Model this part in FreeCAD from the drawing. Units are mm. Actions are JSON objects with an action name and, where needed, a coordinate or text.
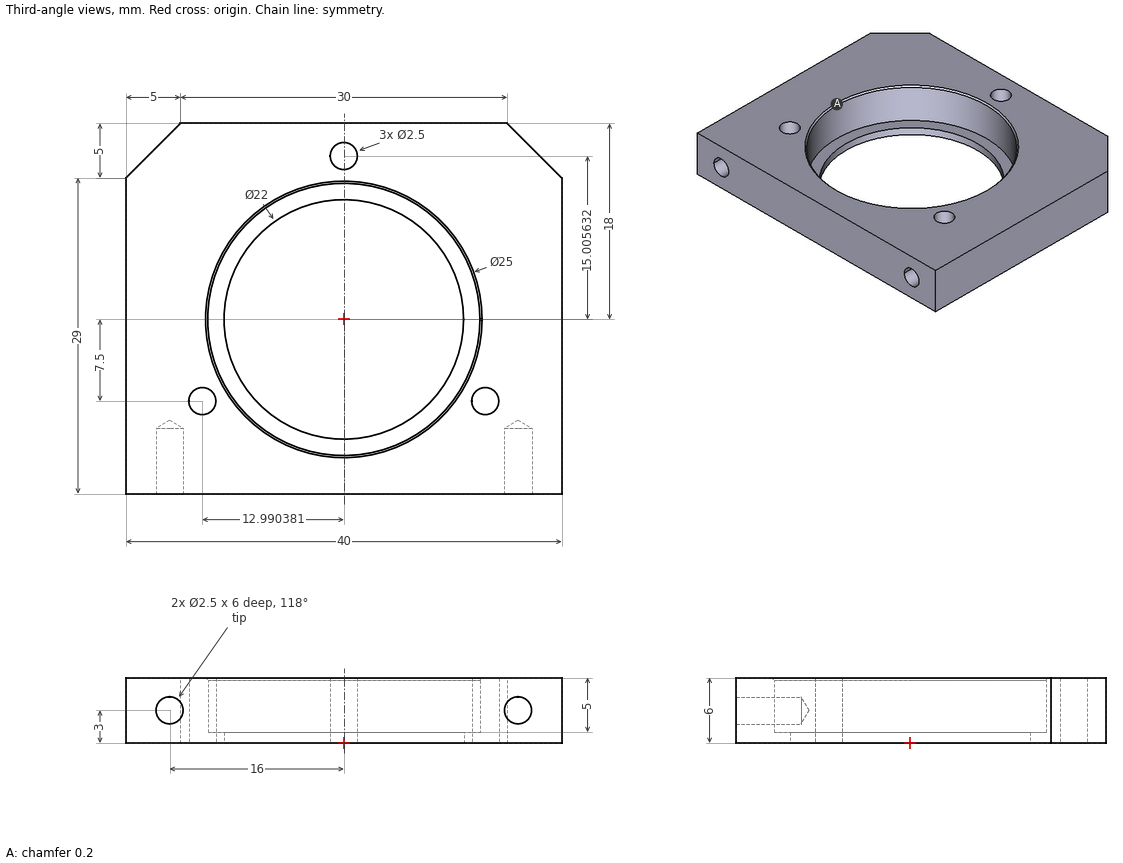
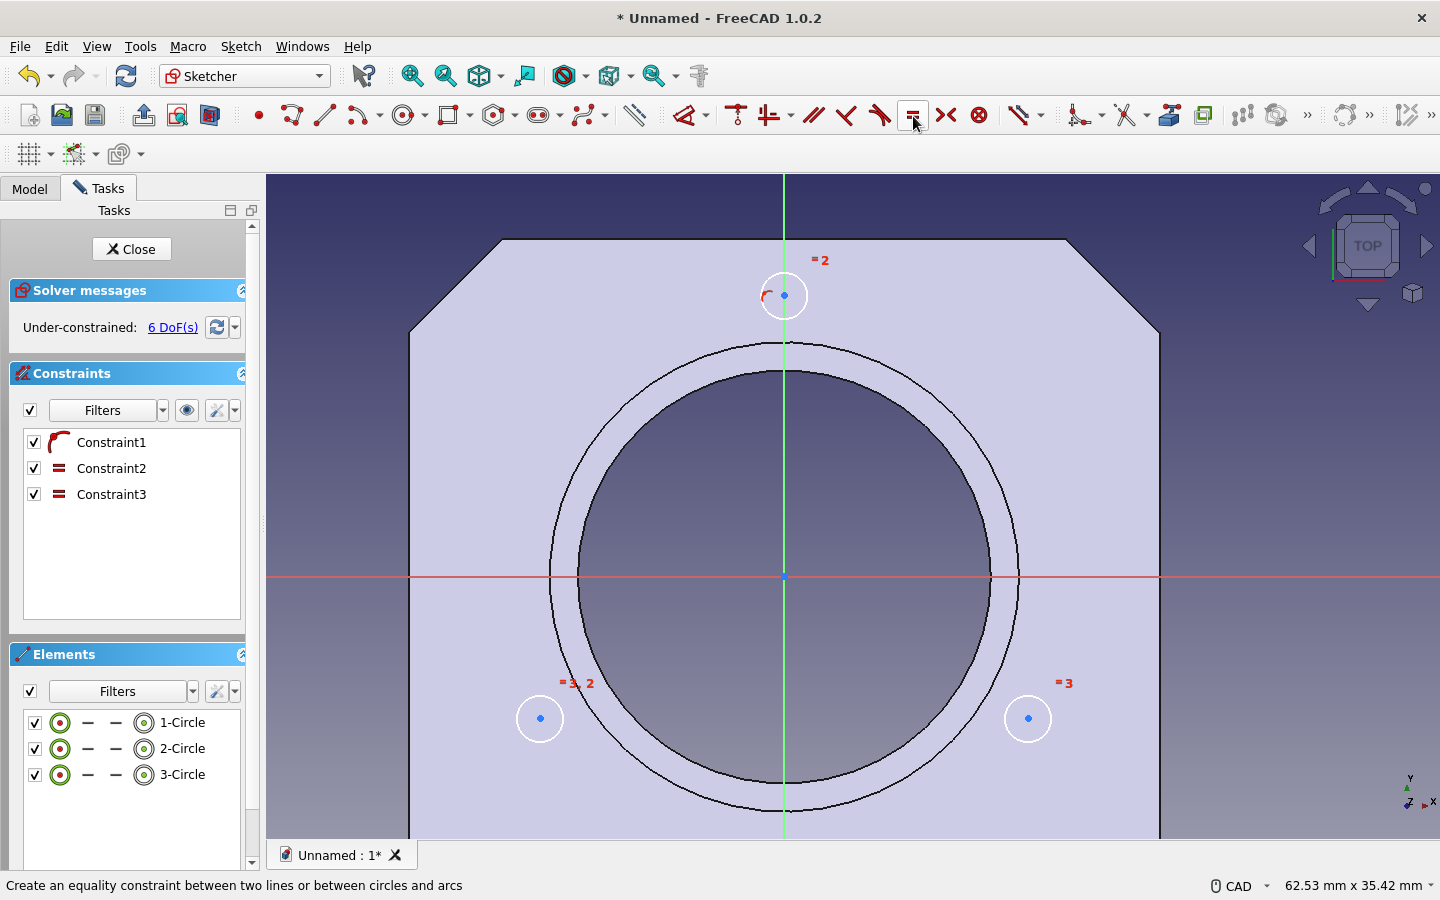
{"action": "left_click", "coordinate": [540, 719]}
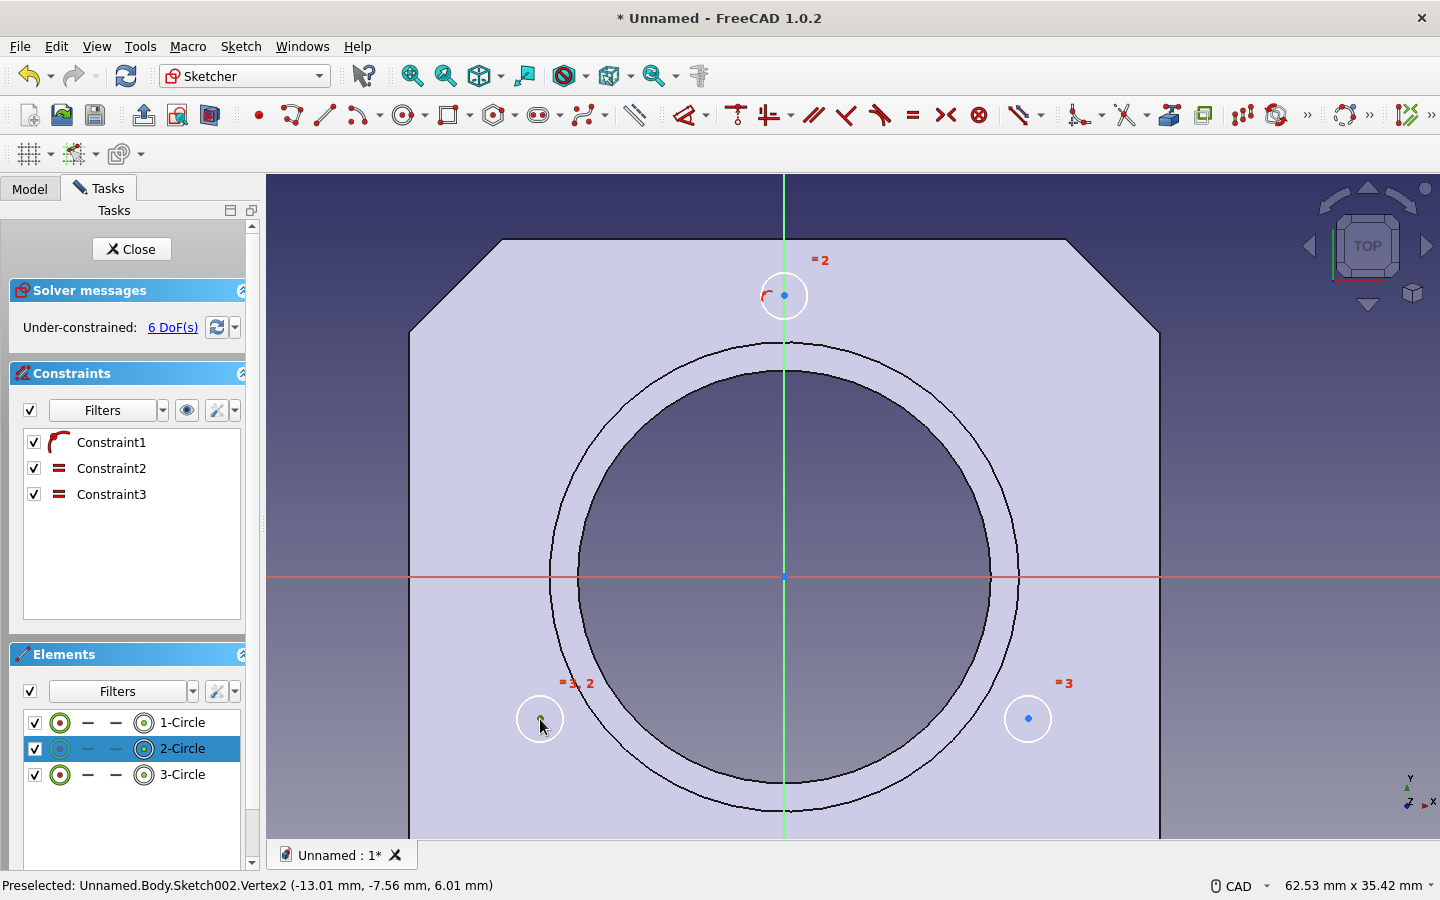
{"action": "left_click", "coordinate": [1028, 719]}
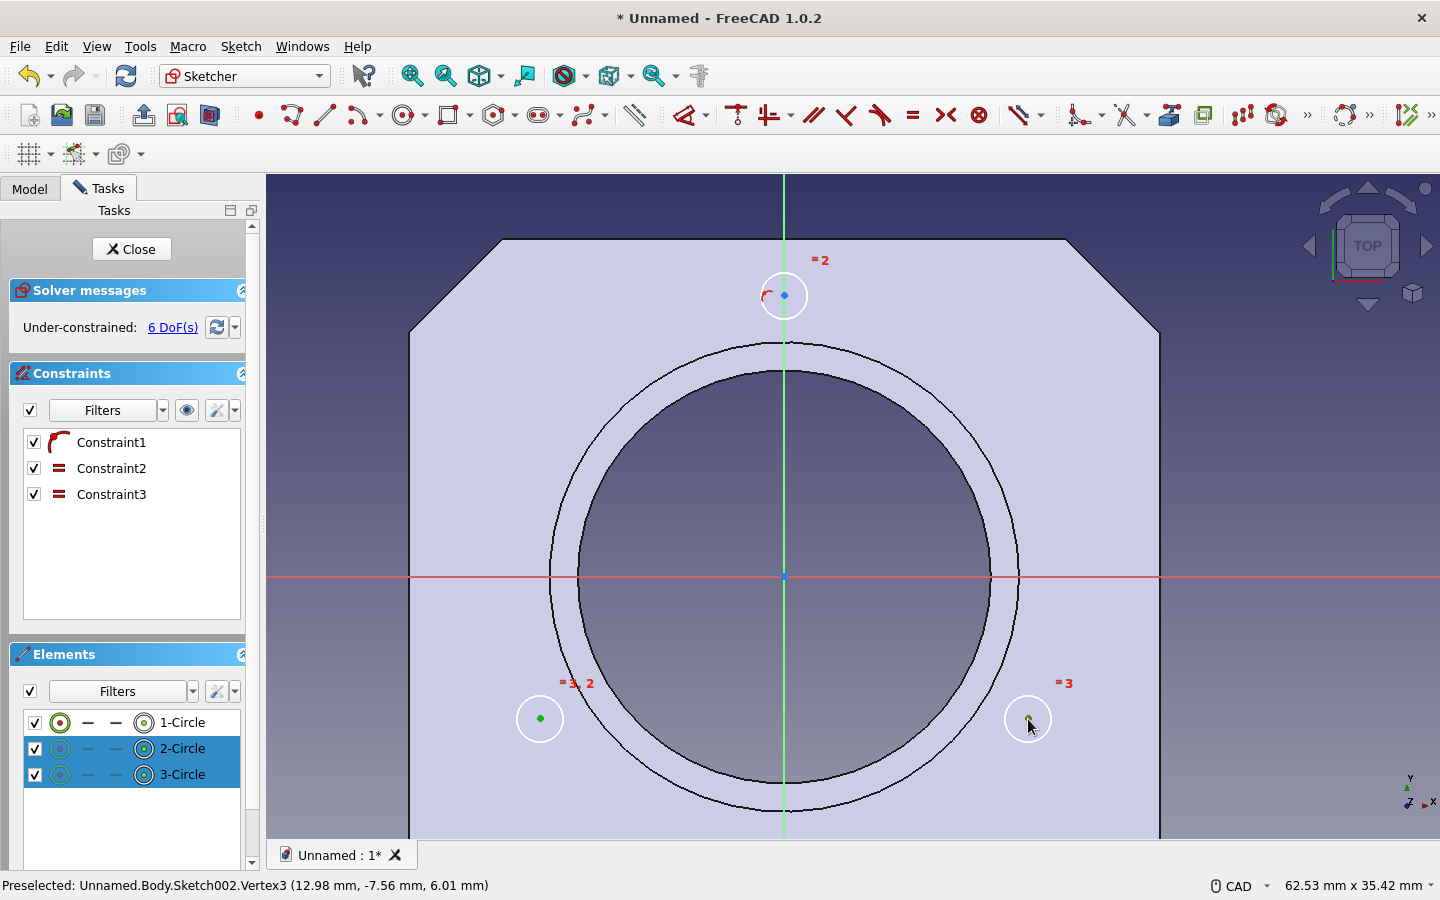
{"action": "left_click", "coordinate": [784, 768]}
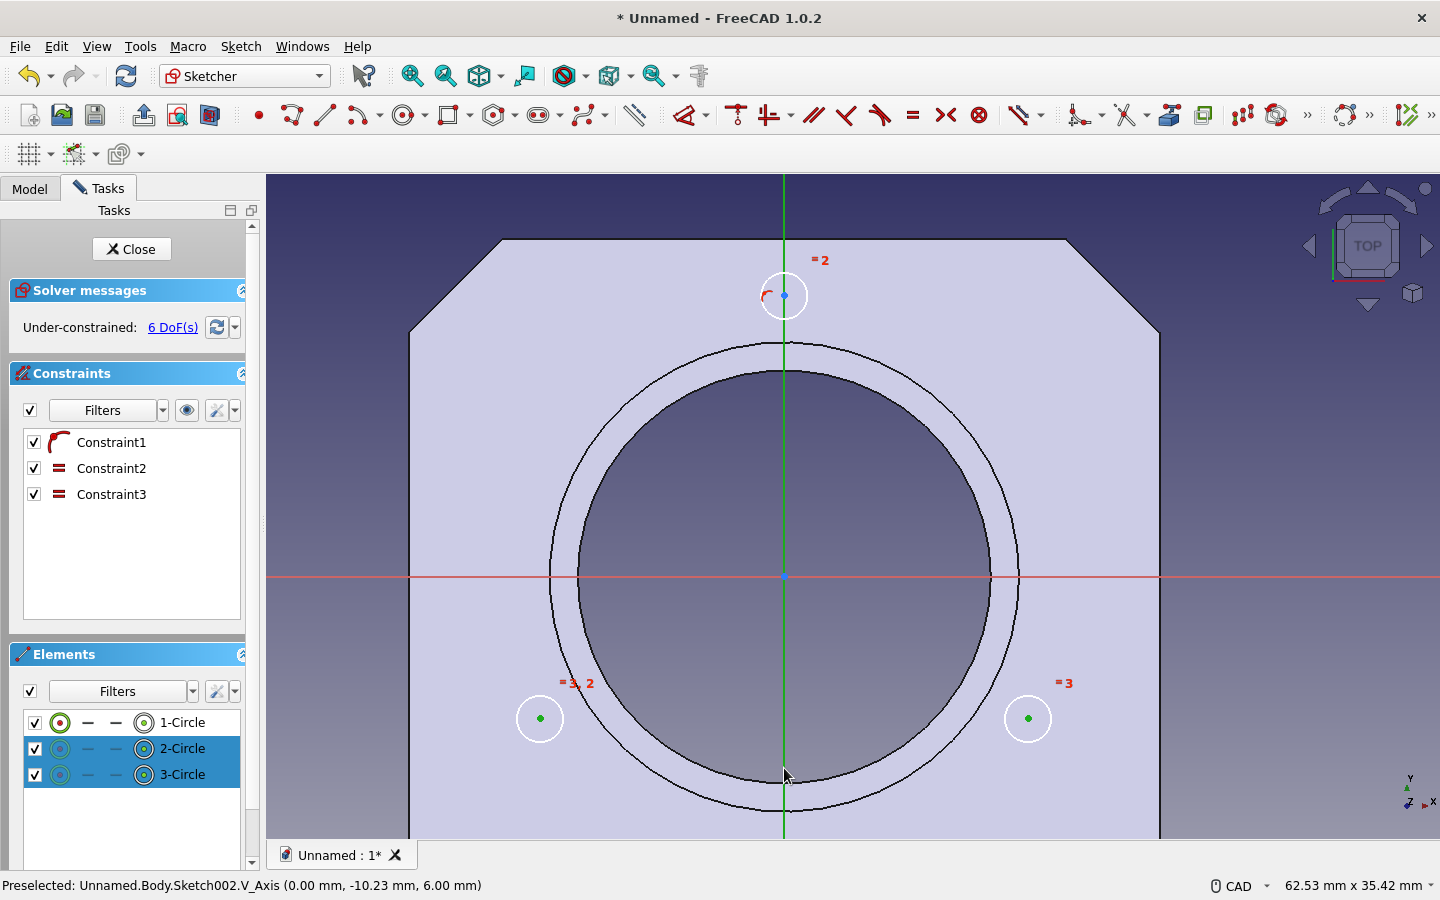
{"action": "key", "text": "s"}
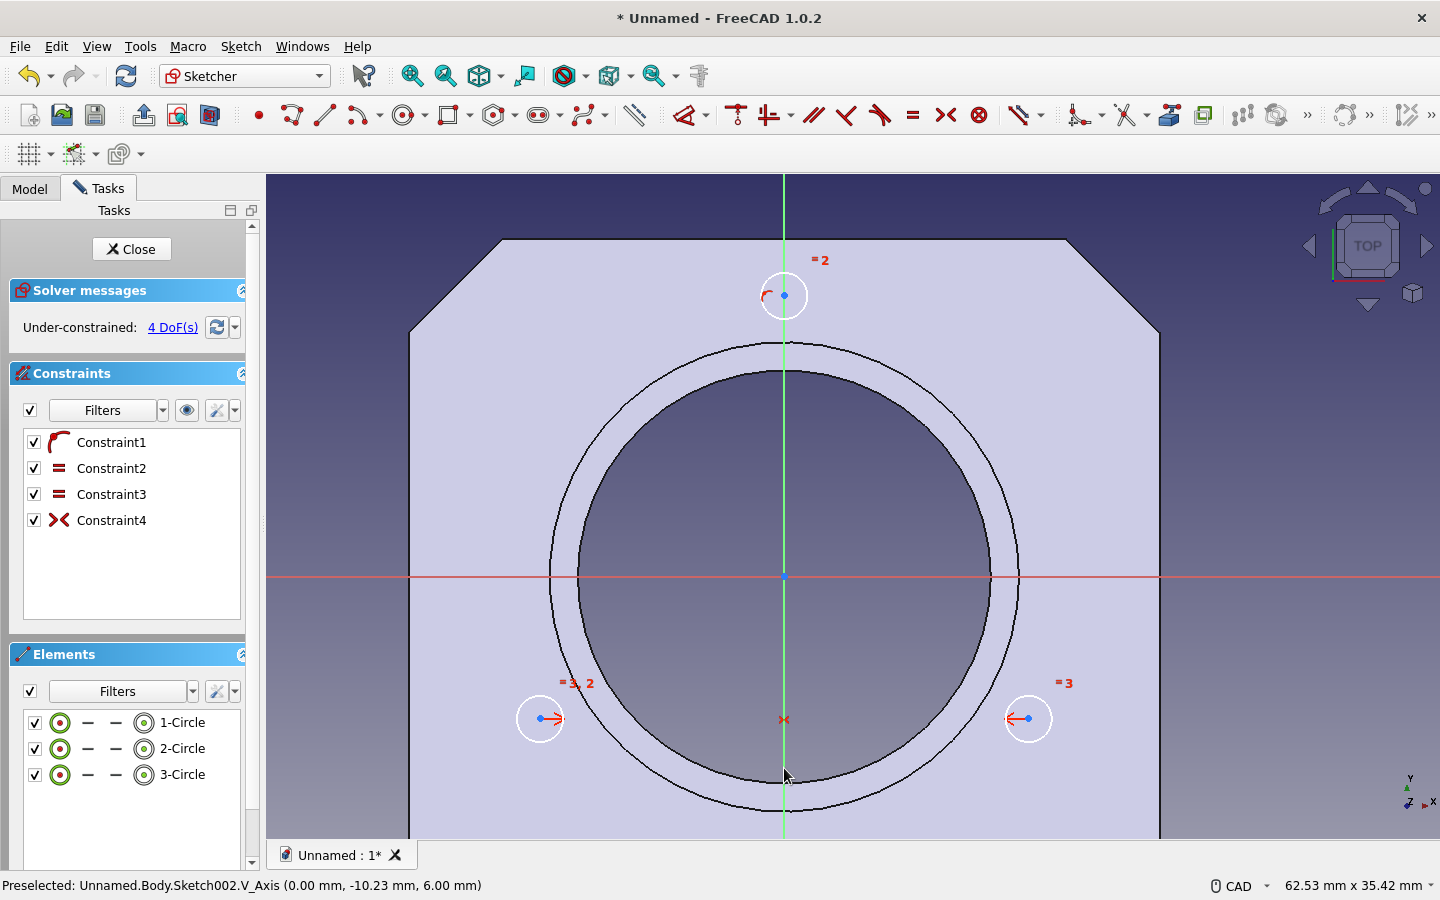
{"action": "key", "text": "d"}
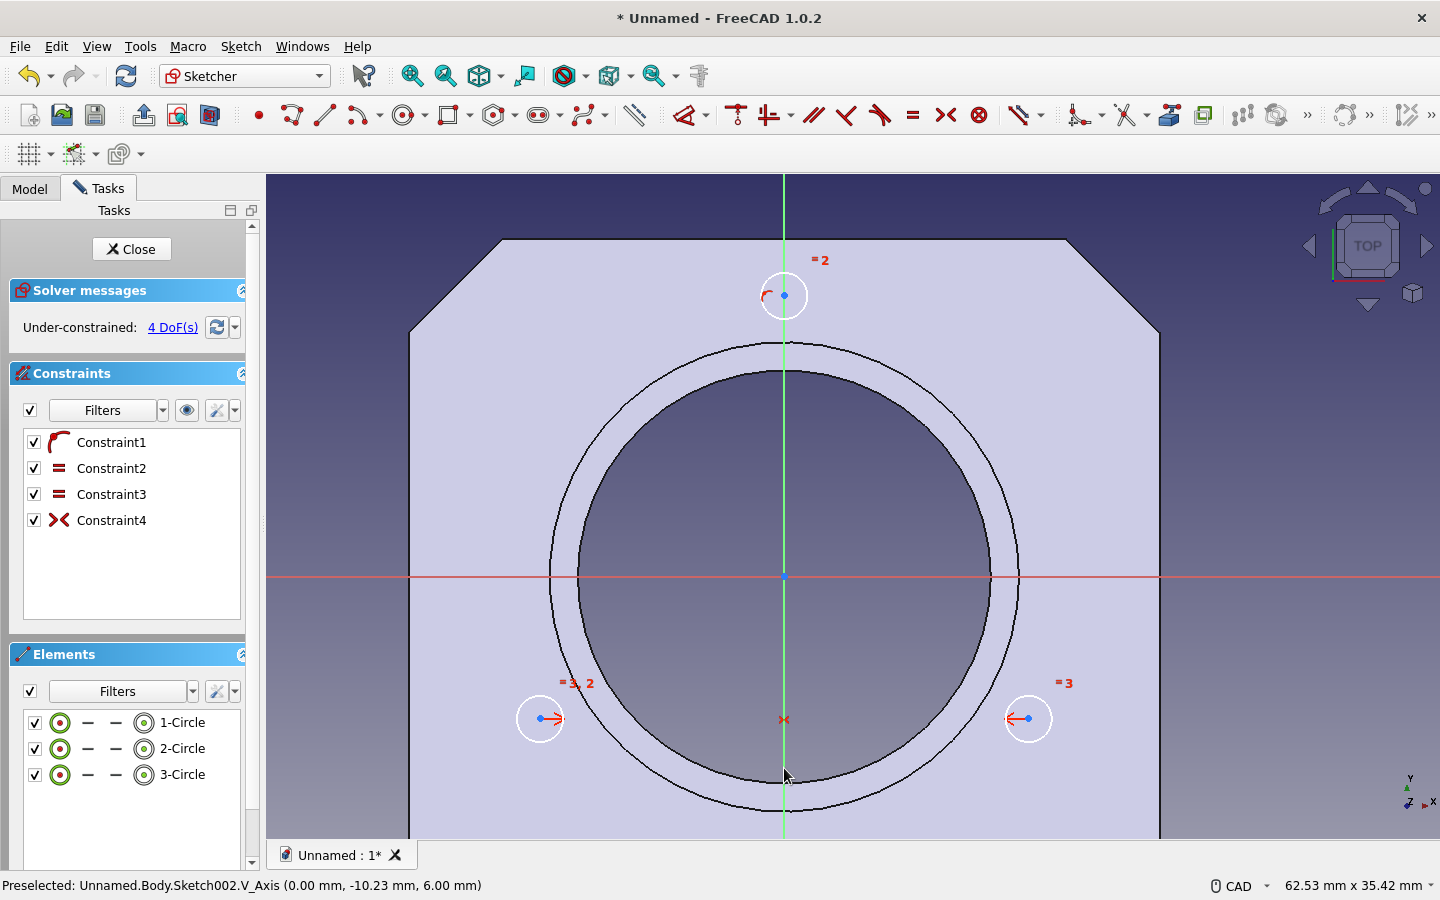
{"action": "left_click", "coordinate": [801, 280]}
{"action": "left_click", "coordinate": [824, 258]}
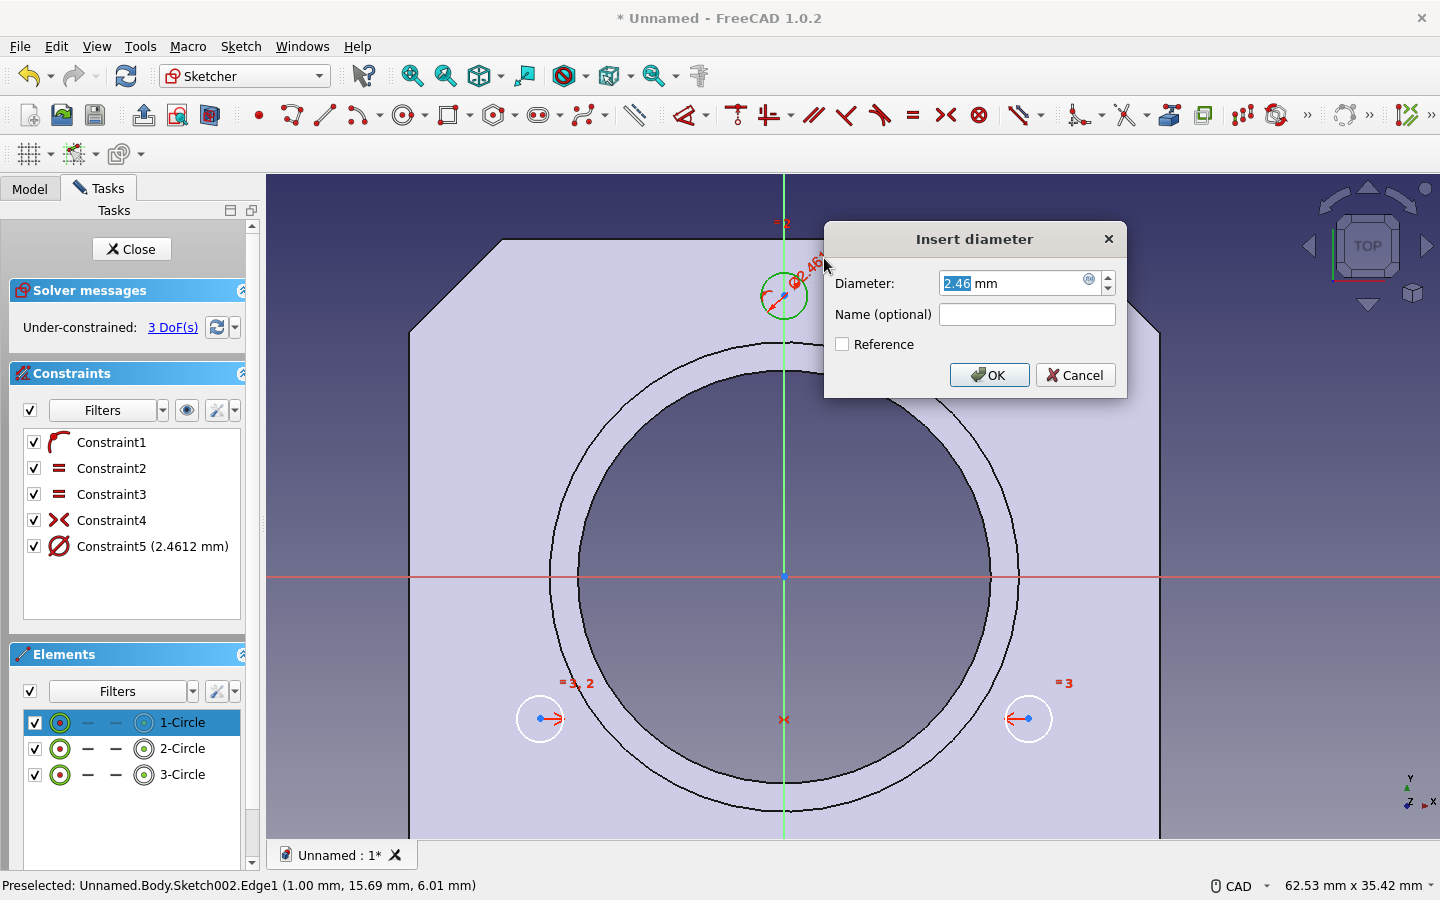
{"action": "type", "text": "2.5"}
{"action": "key", "text": "Return"}